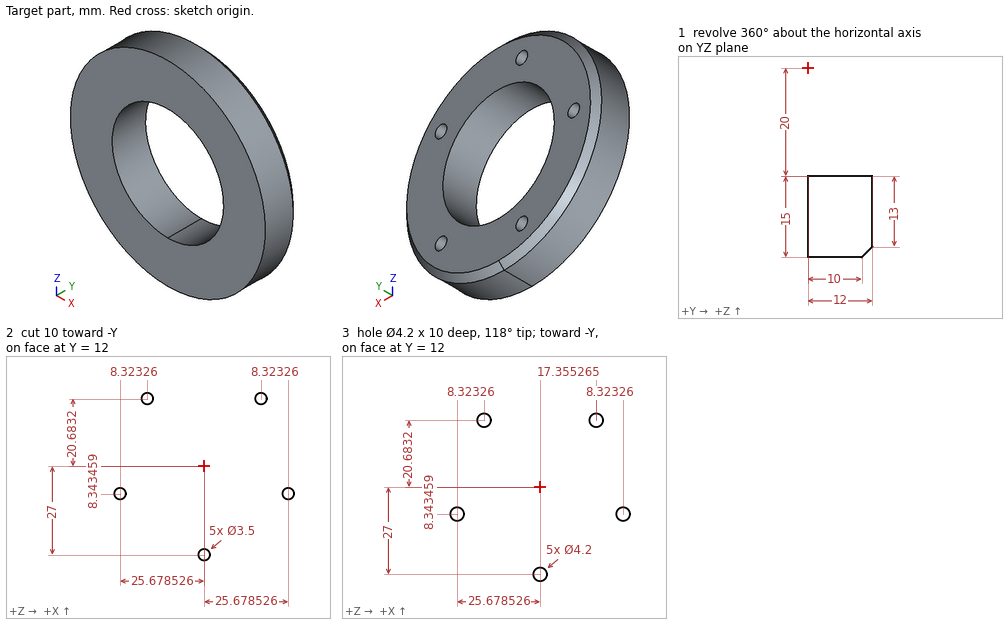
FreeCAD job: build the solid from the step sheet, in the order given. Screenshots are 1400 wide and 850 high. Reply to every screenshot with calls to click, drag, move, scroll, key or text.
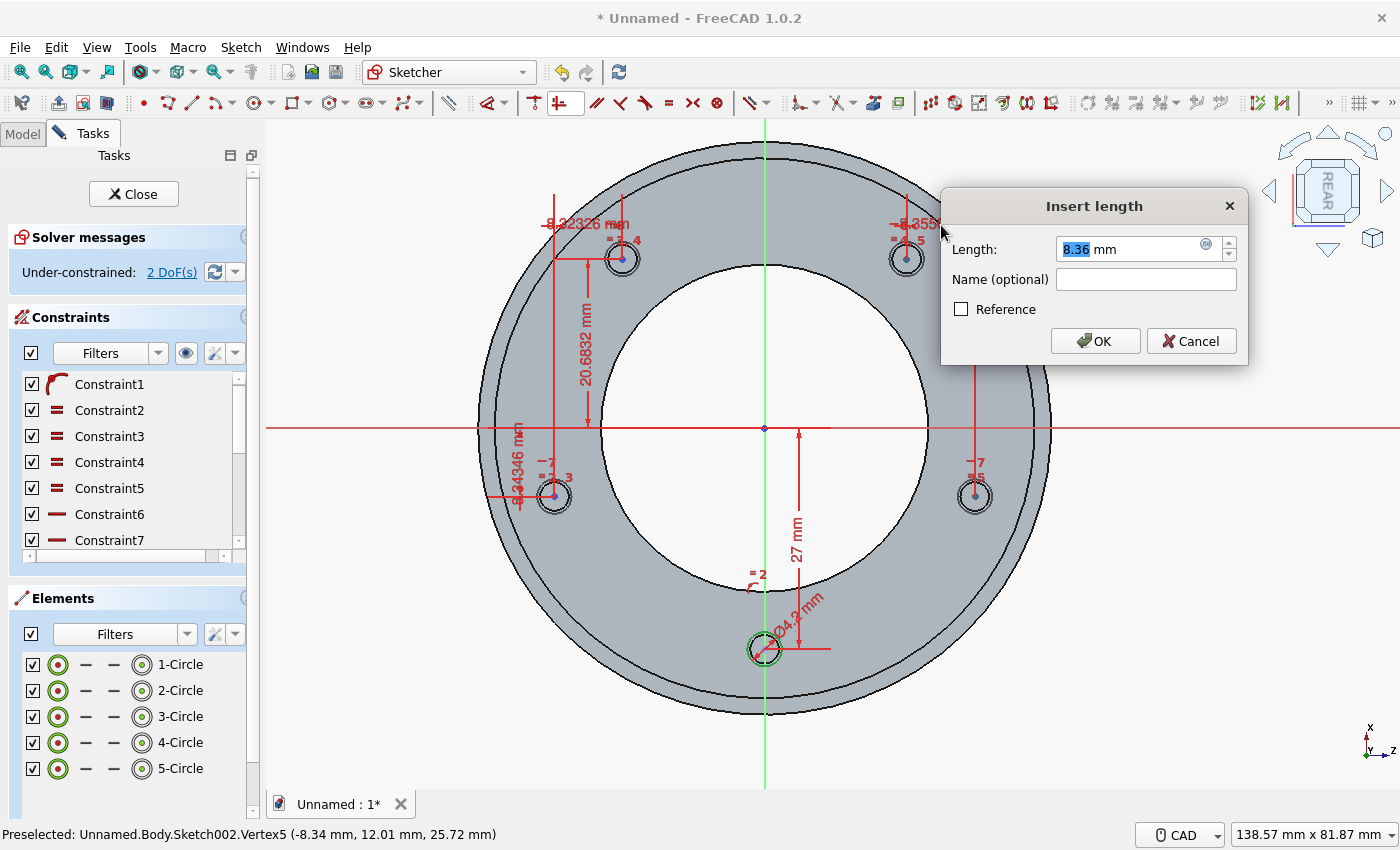
text(8.32326)
key(Return)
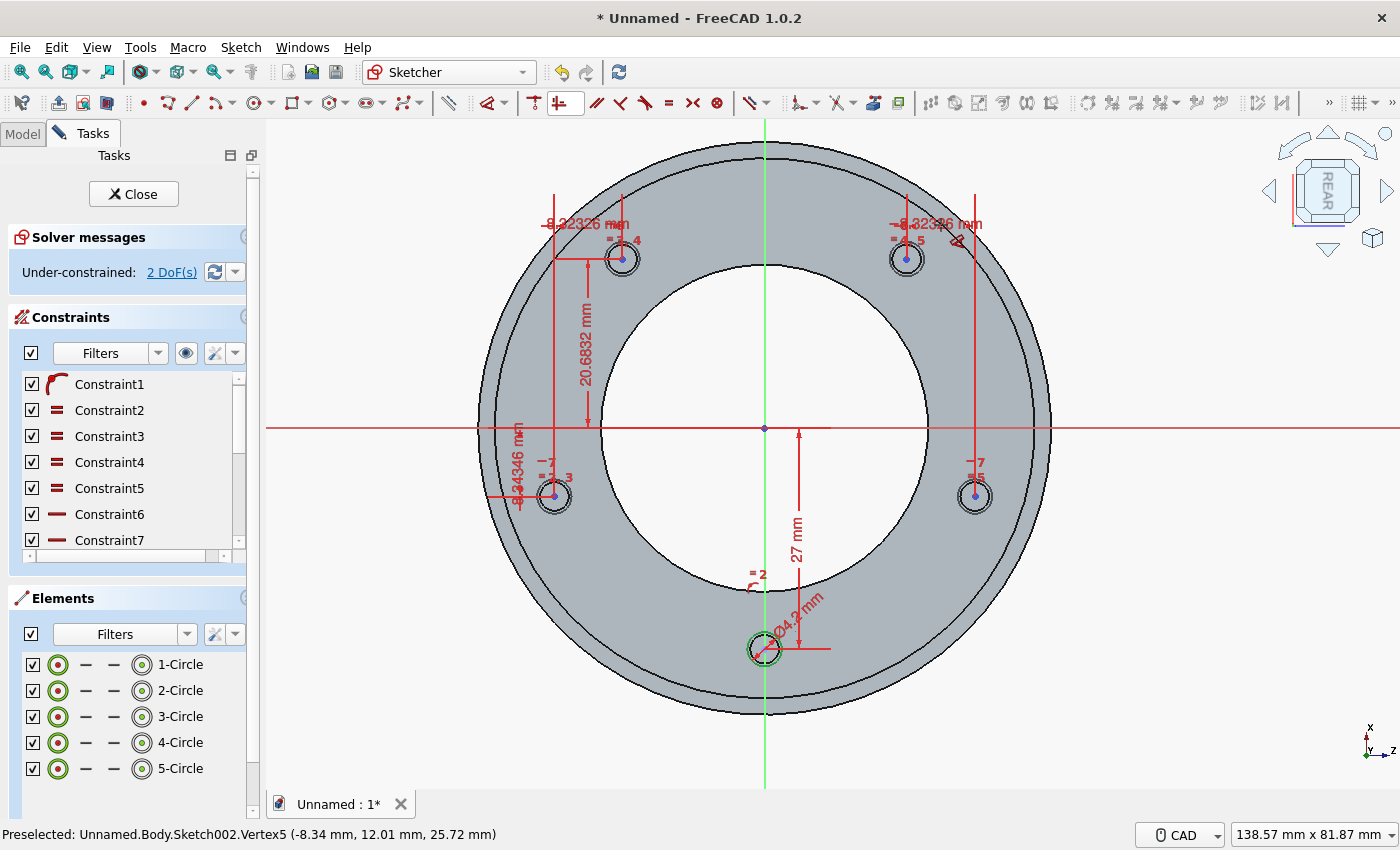
click(554, 497)
click(659, 531)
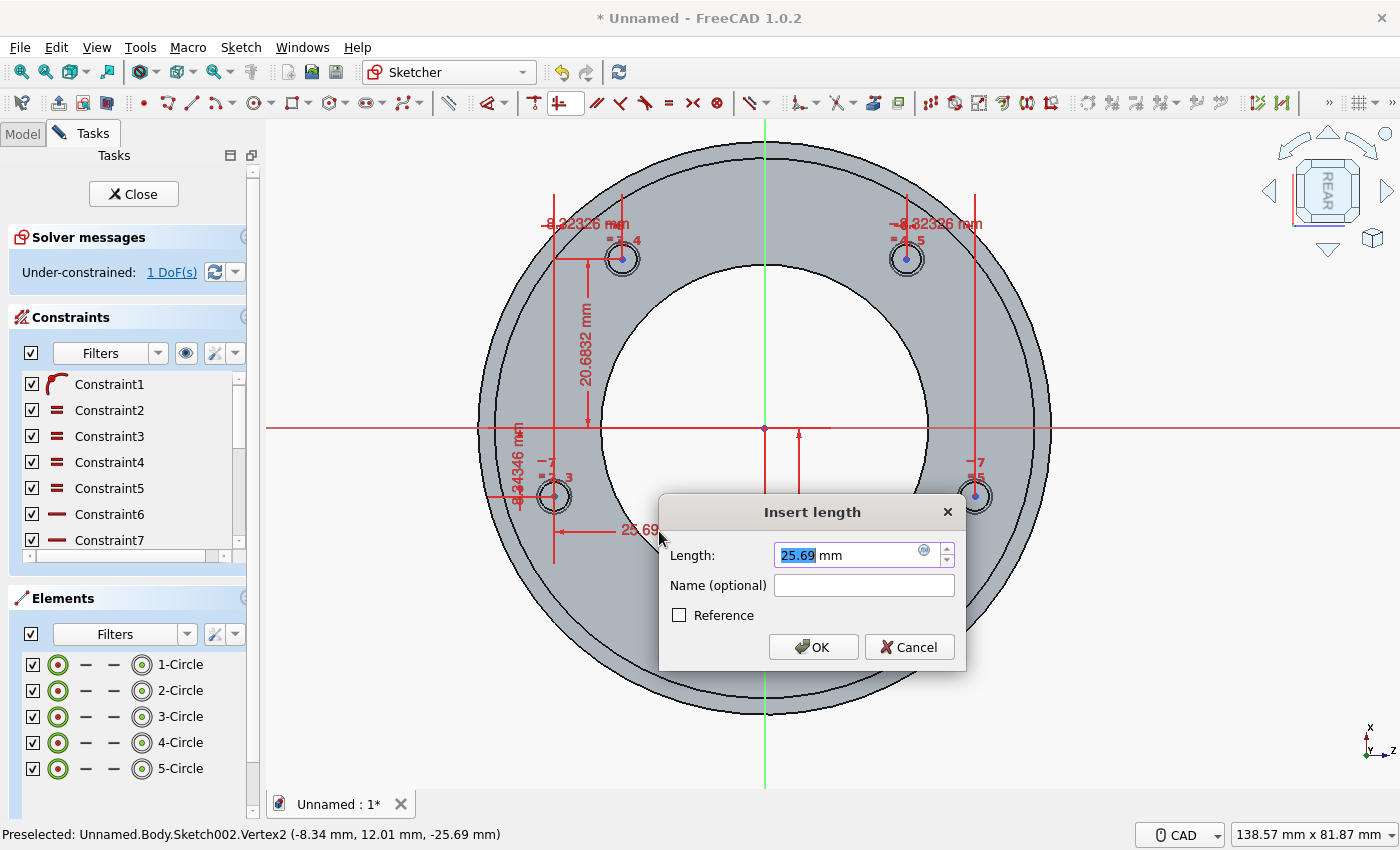
text(25.678526)
key(Return)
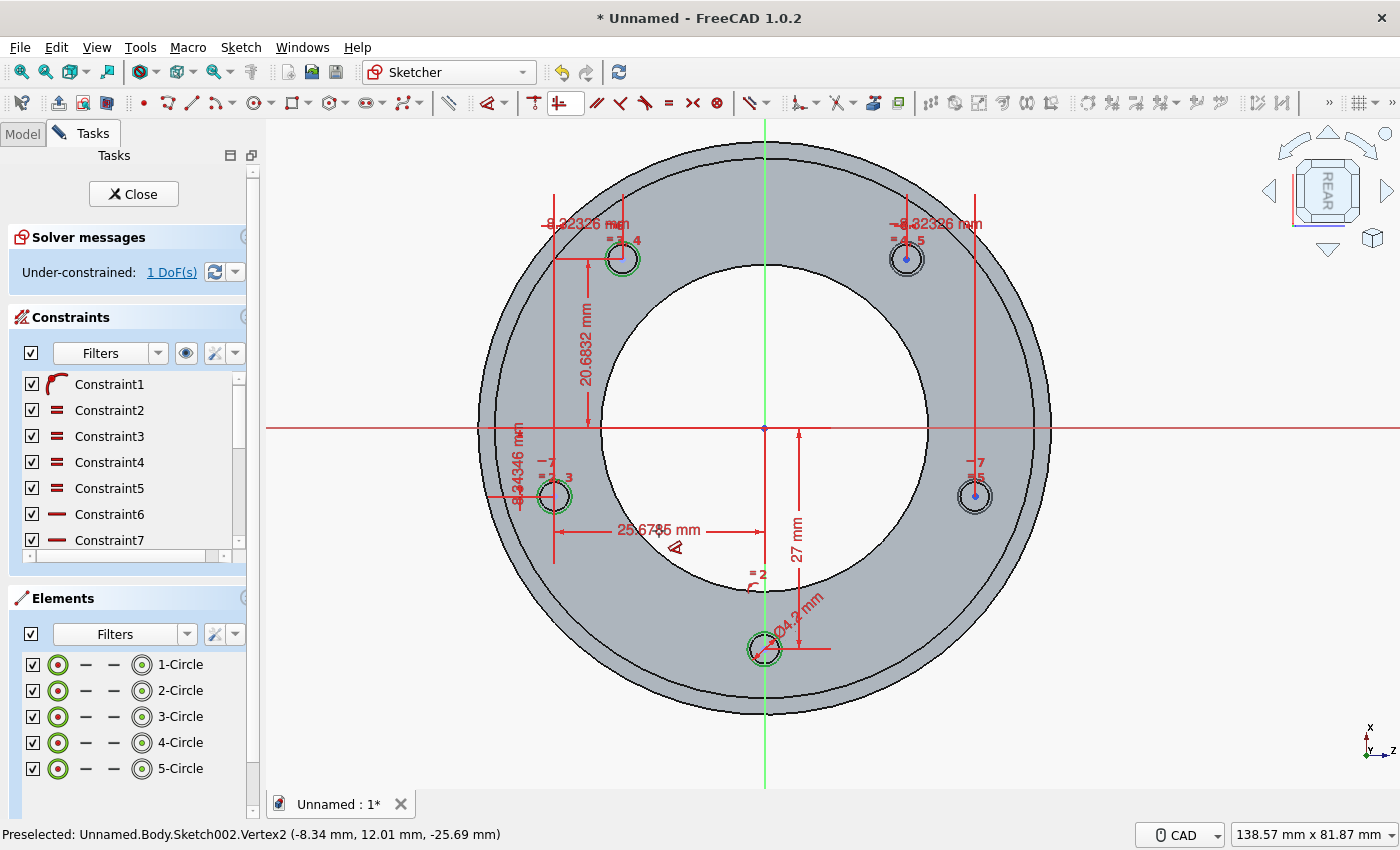
click(907, 259)
click(836, 225)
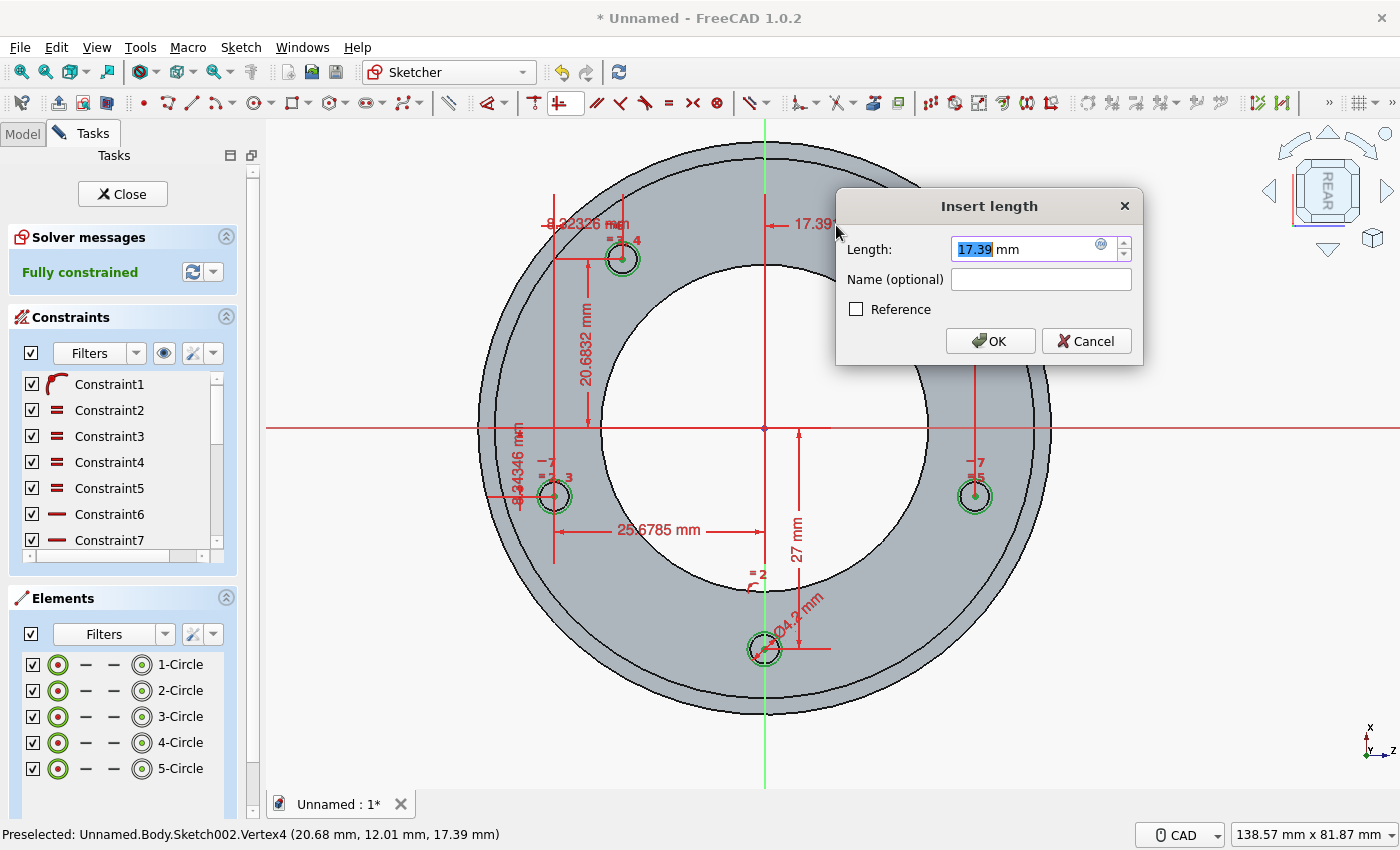
text(17.355265)
key(Return)
key(Escape)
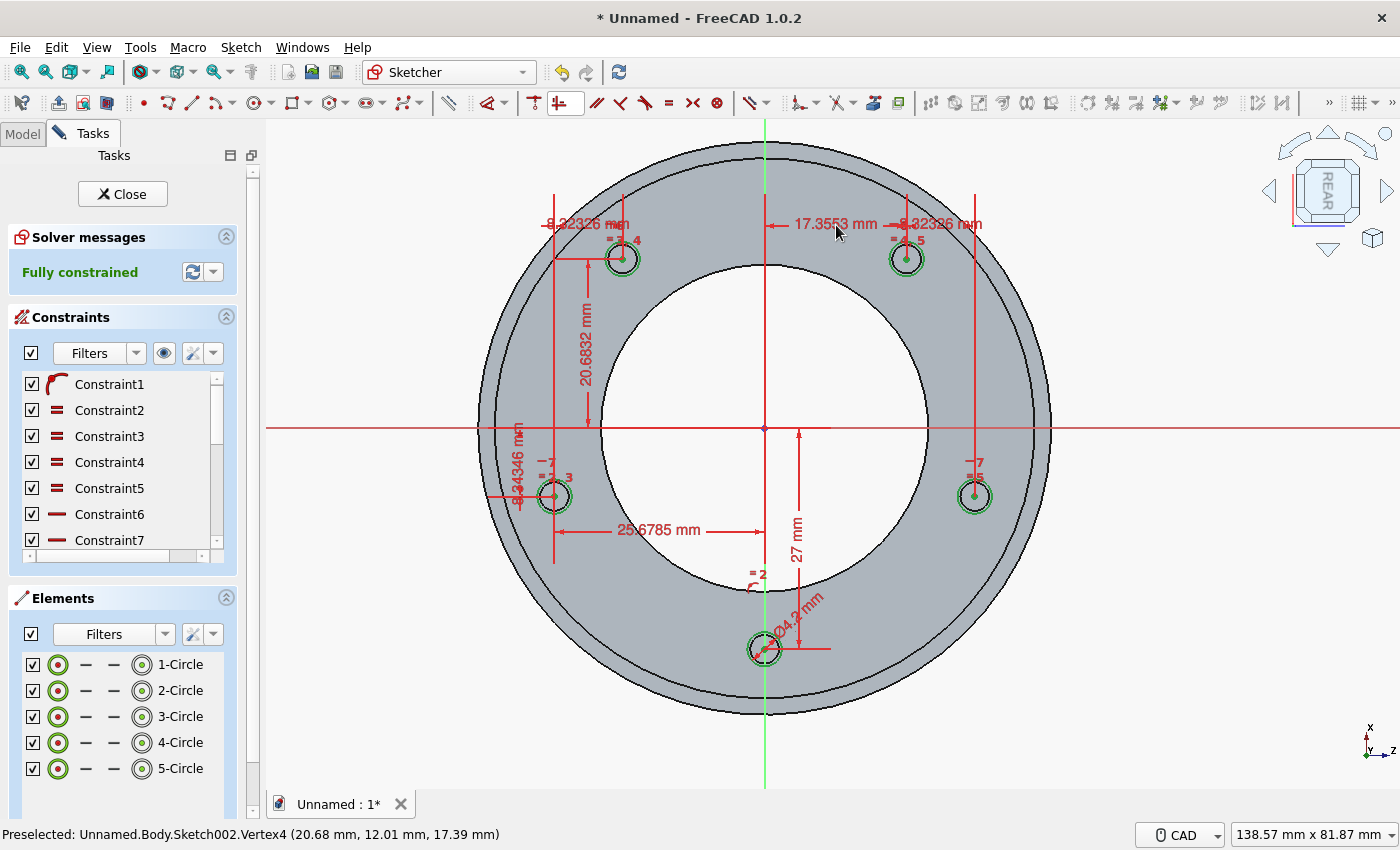
click(123, 194)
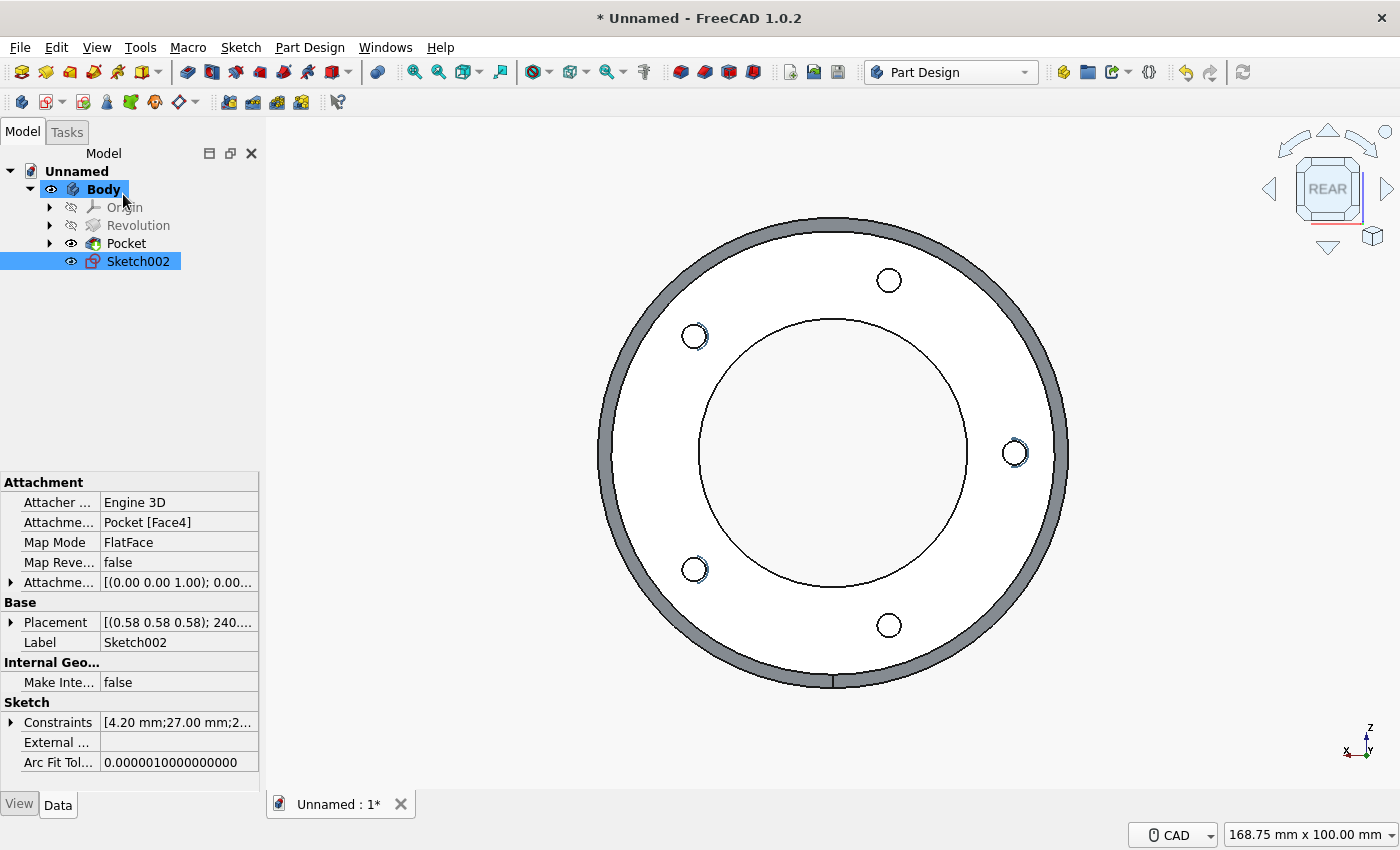
click(212, 72)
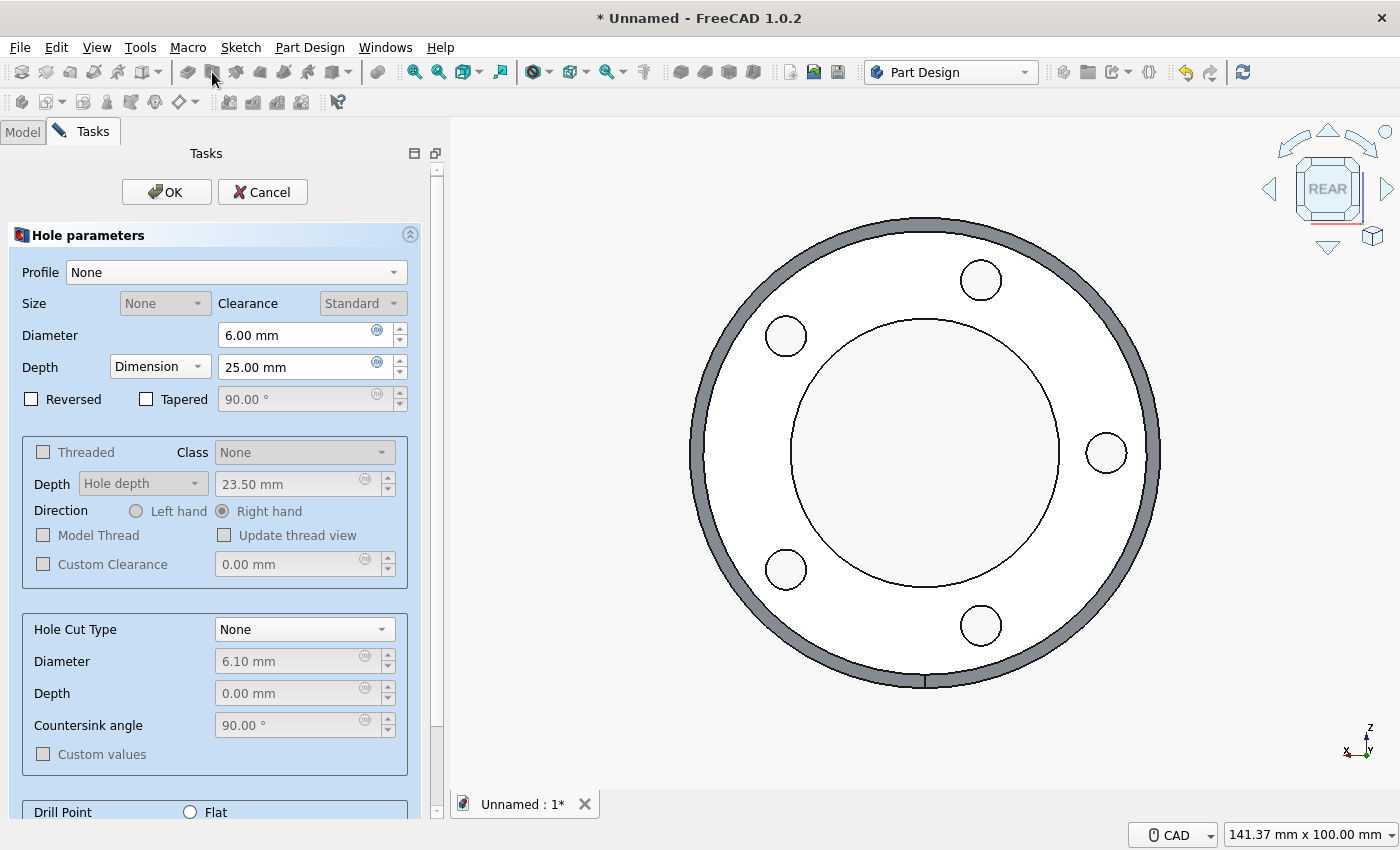
triple_click(305, 335)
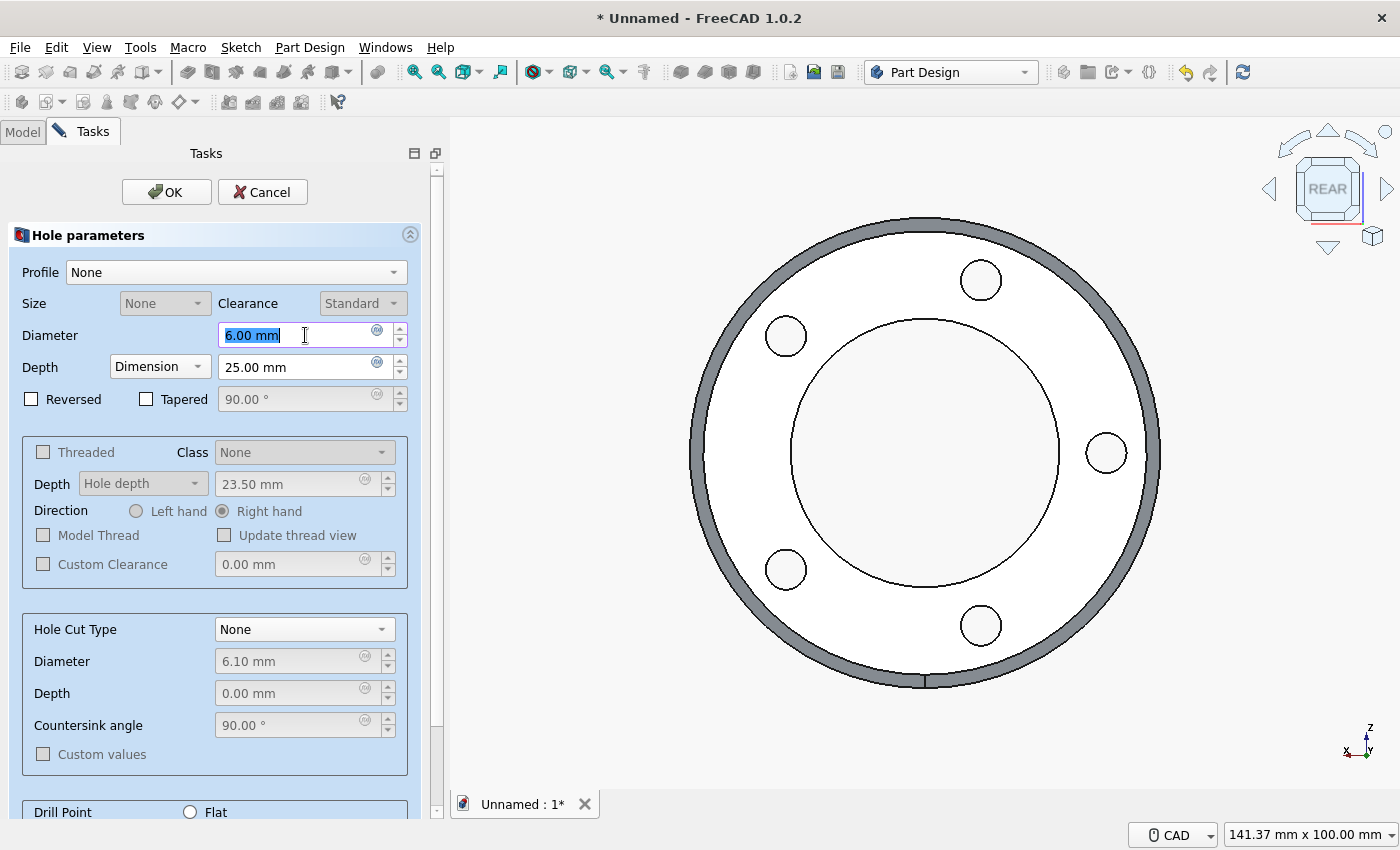
text(4.2)
key(Tab)